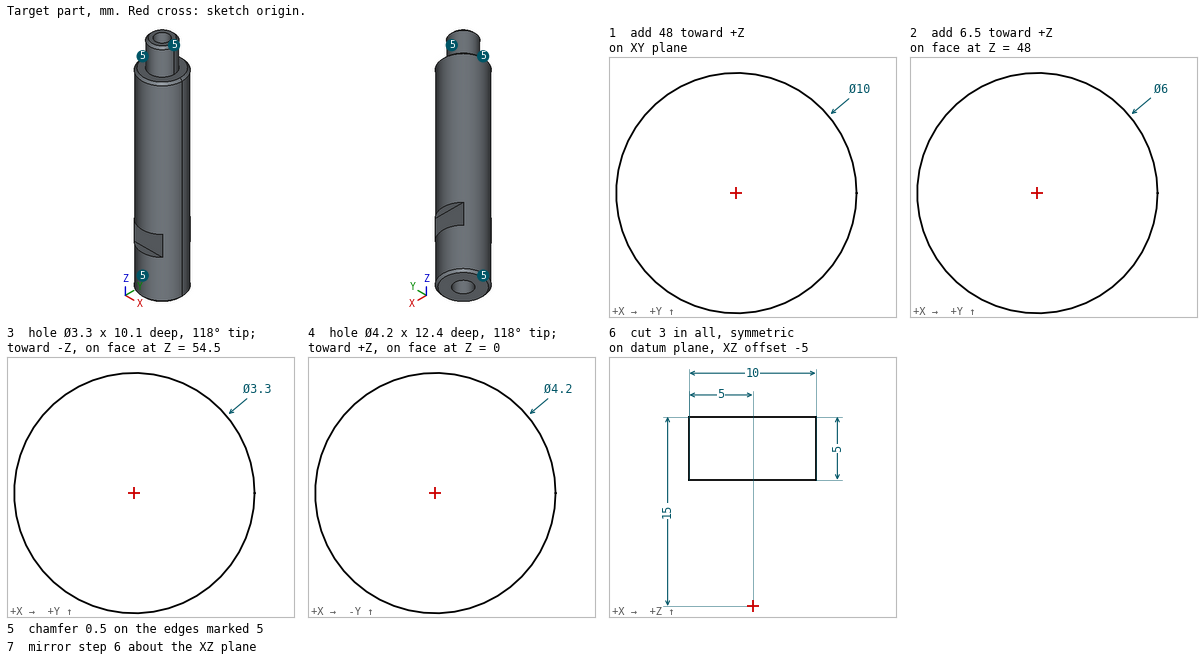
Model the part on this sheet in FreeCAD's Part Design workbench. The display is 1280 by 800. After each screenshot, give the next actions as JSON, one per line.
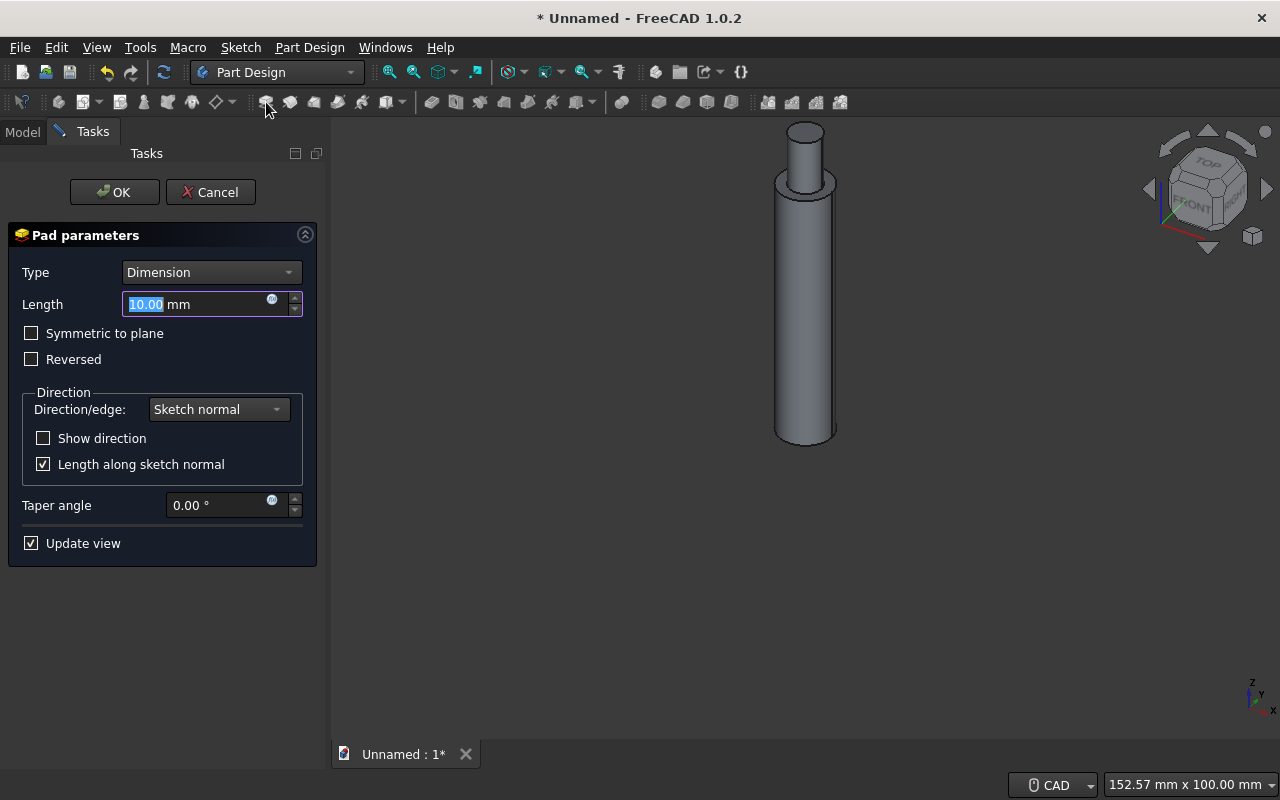
{"action": "type", "text": "6.5"}
{"action": "key", "text": "Tab"}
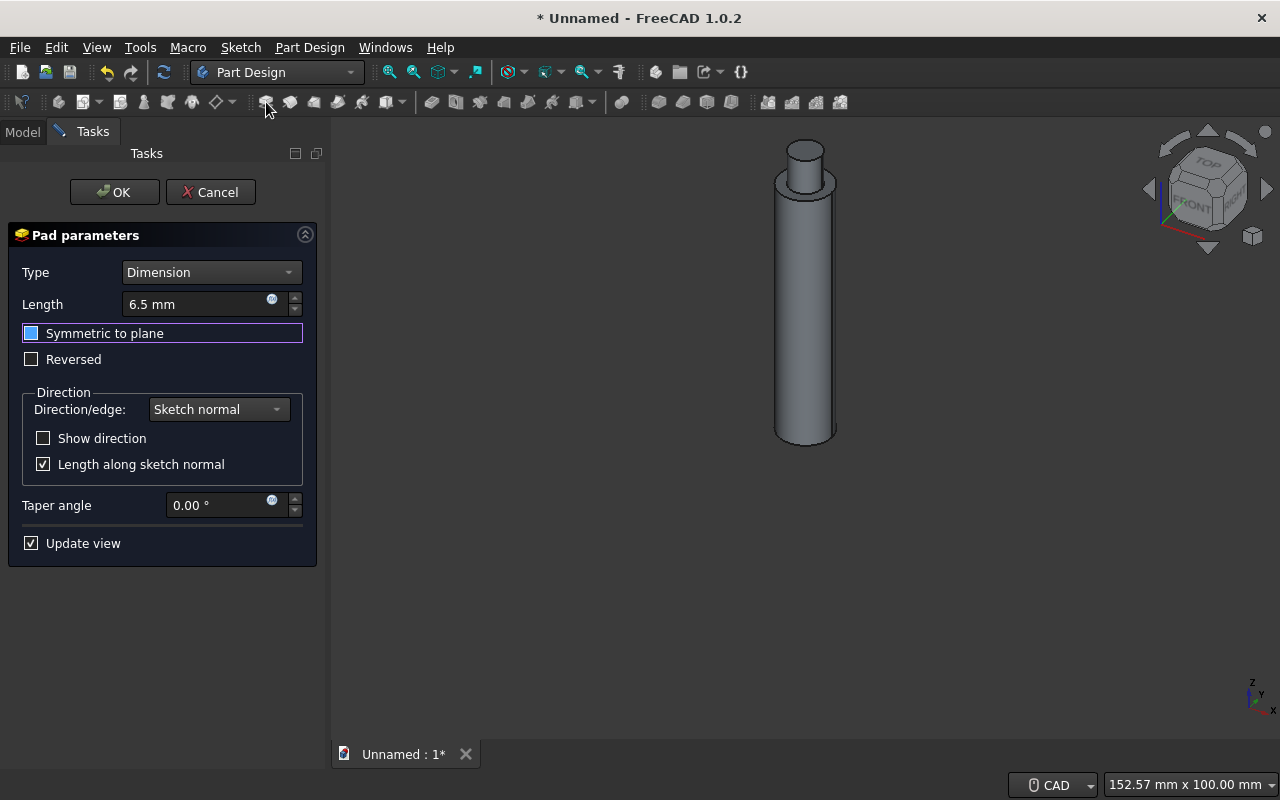
{"action": "left_click", "coordinate": [115, 192]}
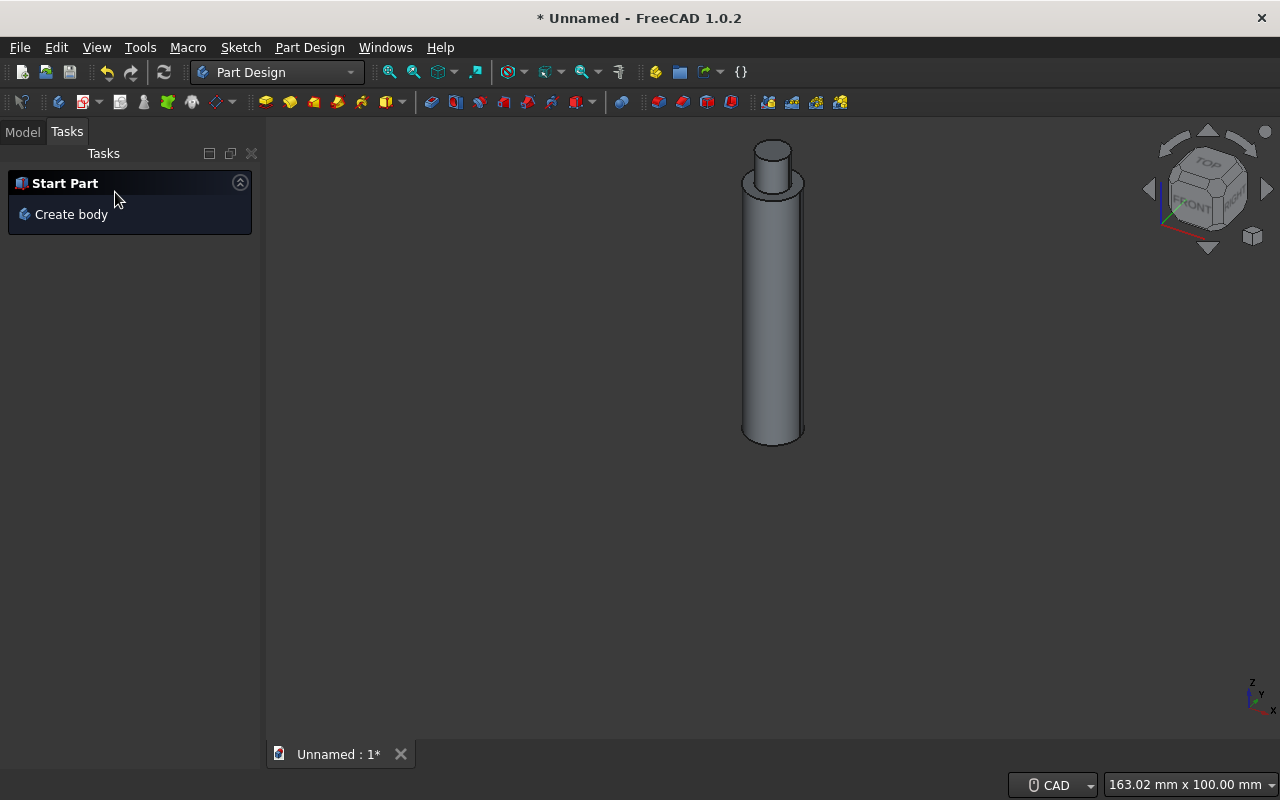
{"action": "left_click", "coordinate": [773, 149]}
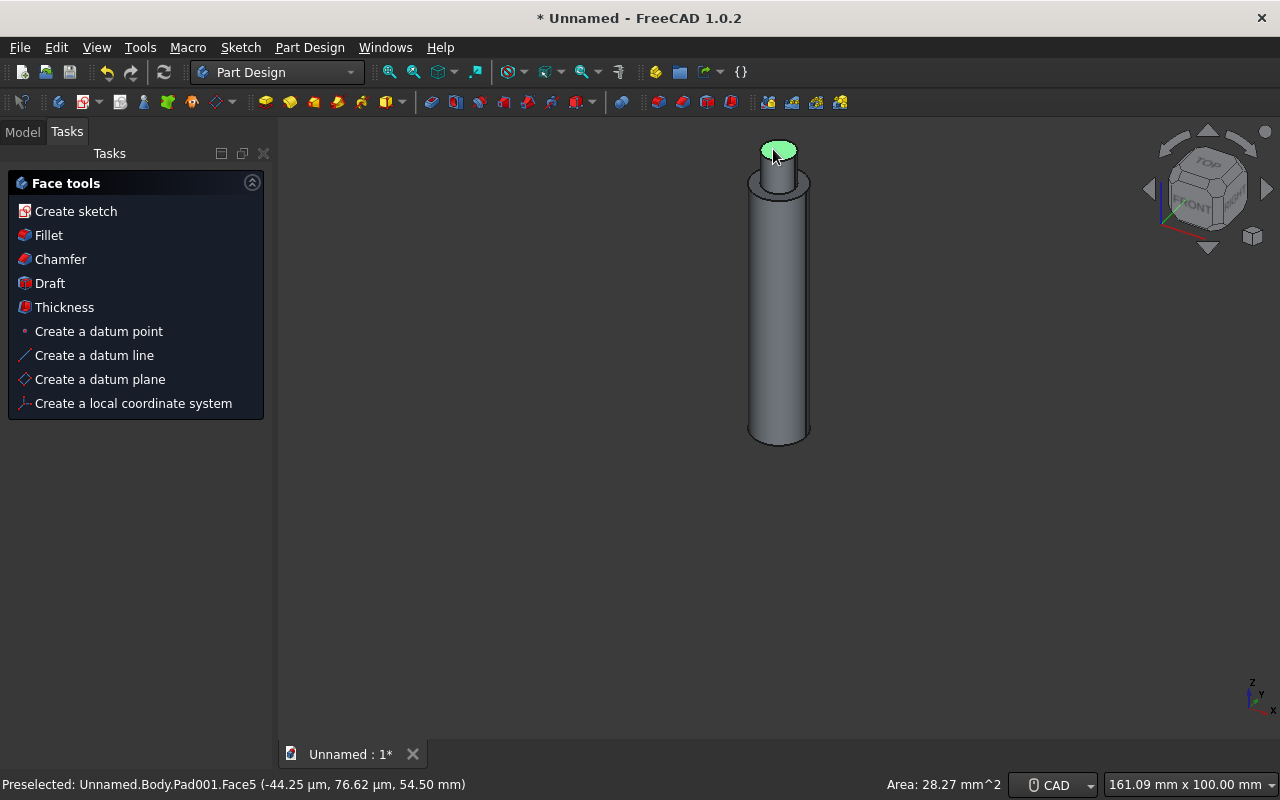
{"action": "left_click", "coordinate": [84, 102]}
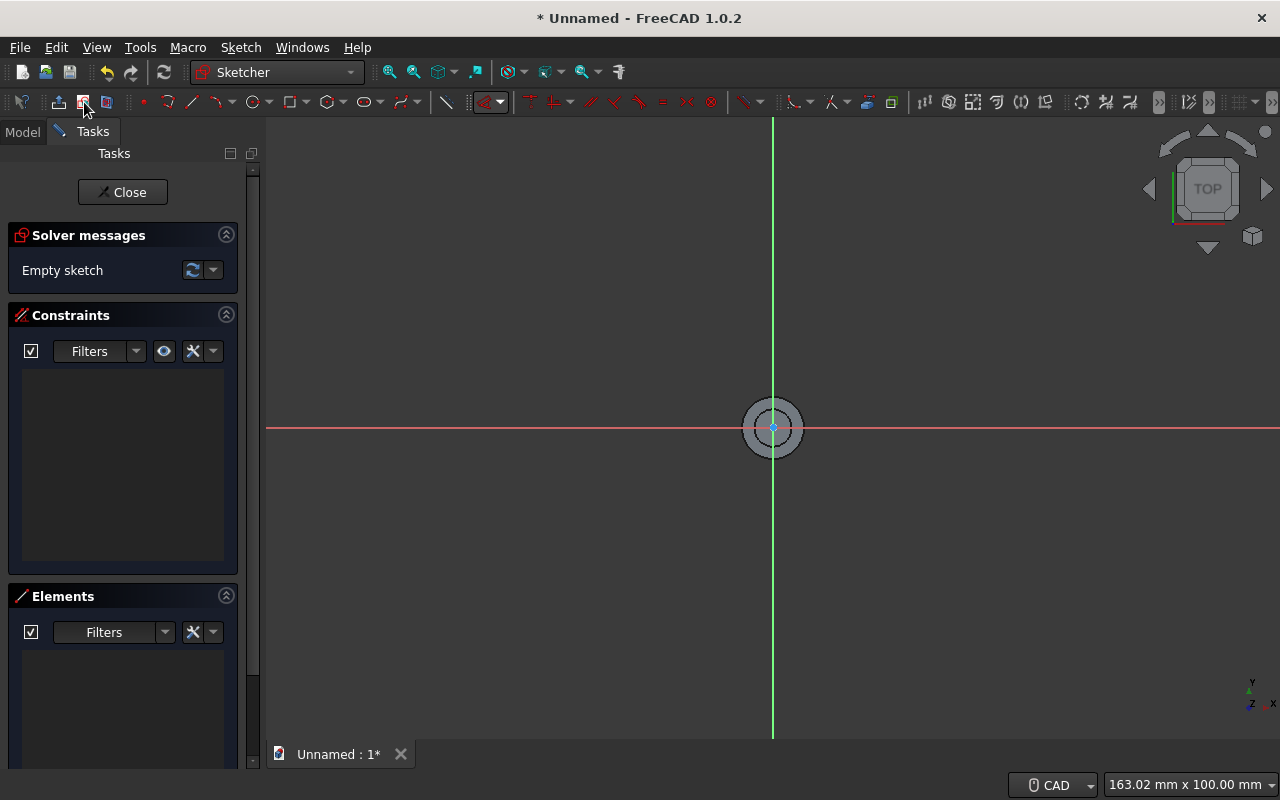
{"action": "scroll", "coordinate": [777, 428], "scroll_direction": "up", "scroll_amount": 15}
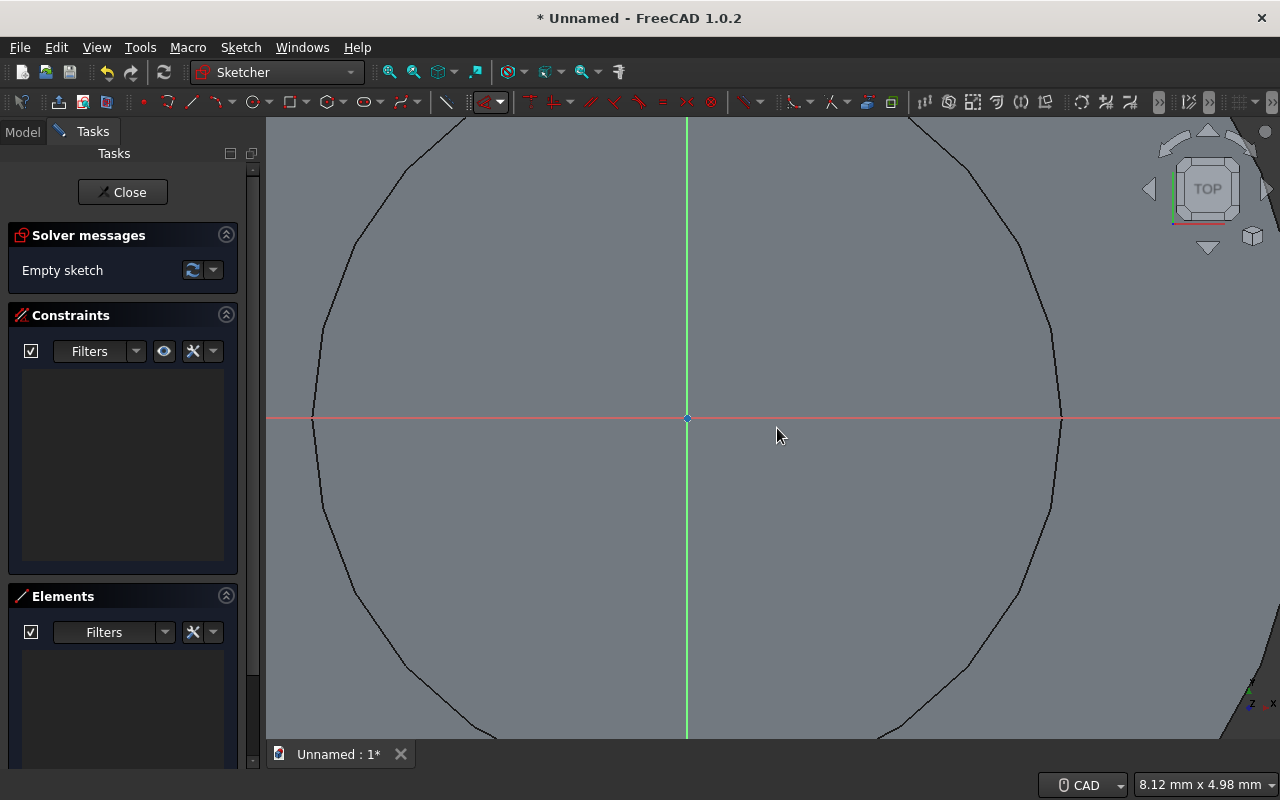
{"action": "left_click", "coordinate": [254, 102]}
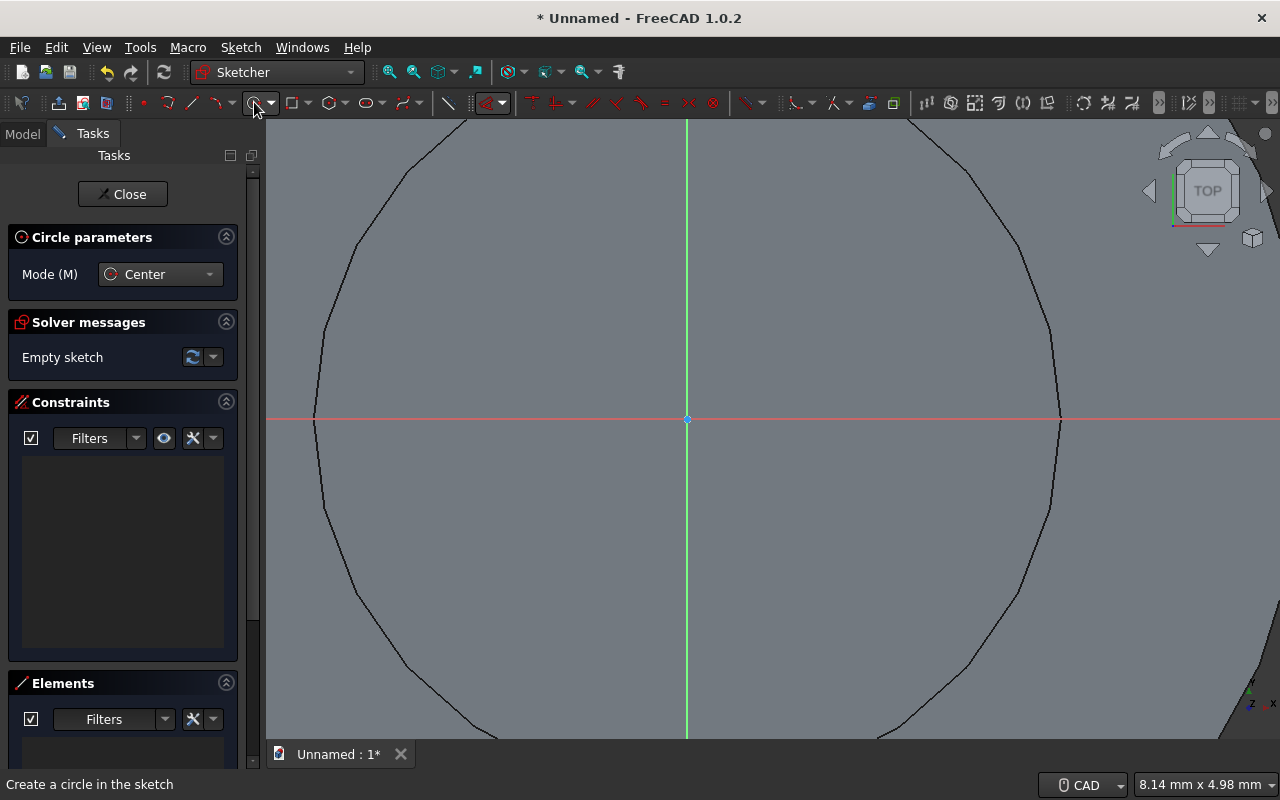
{"action": "left_click", "coordinate": [687, 419]}
{"action": "mouse_move", "coordinate": [833, 274]}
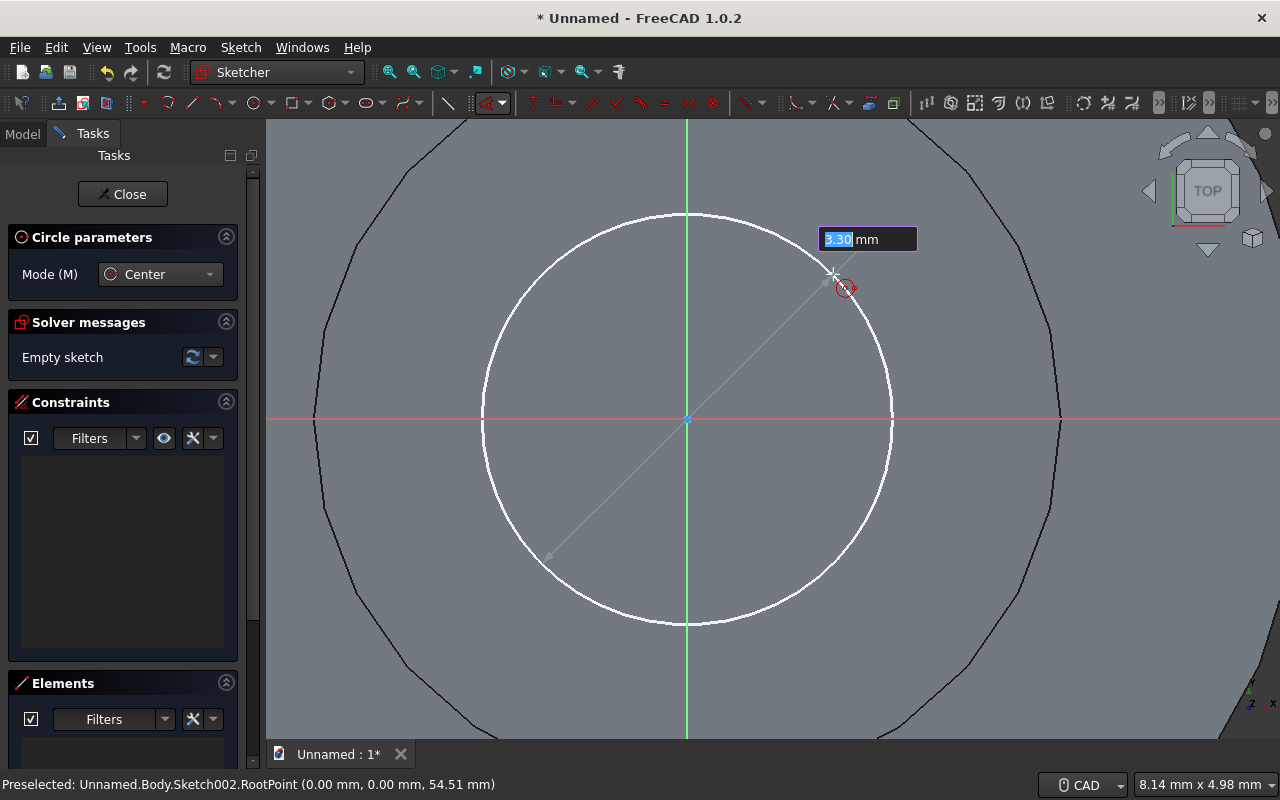
{"action": "type", "text": "3.3"}
{"action": "key", "text": "Return"}
{"action": "key", "text": "Escape"}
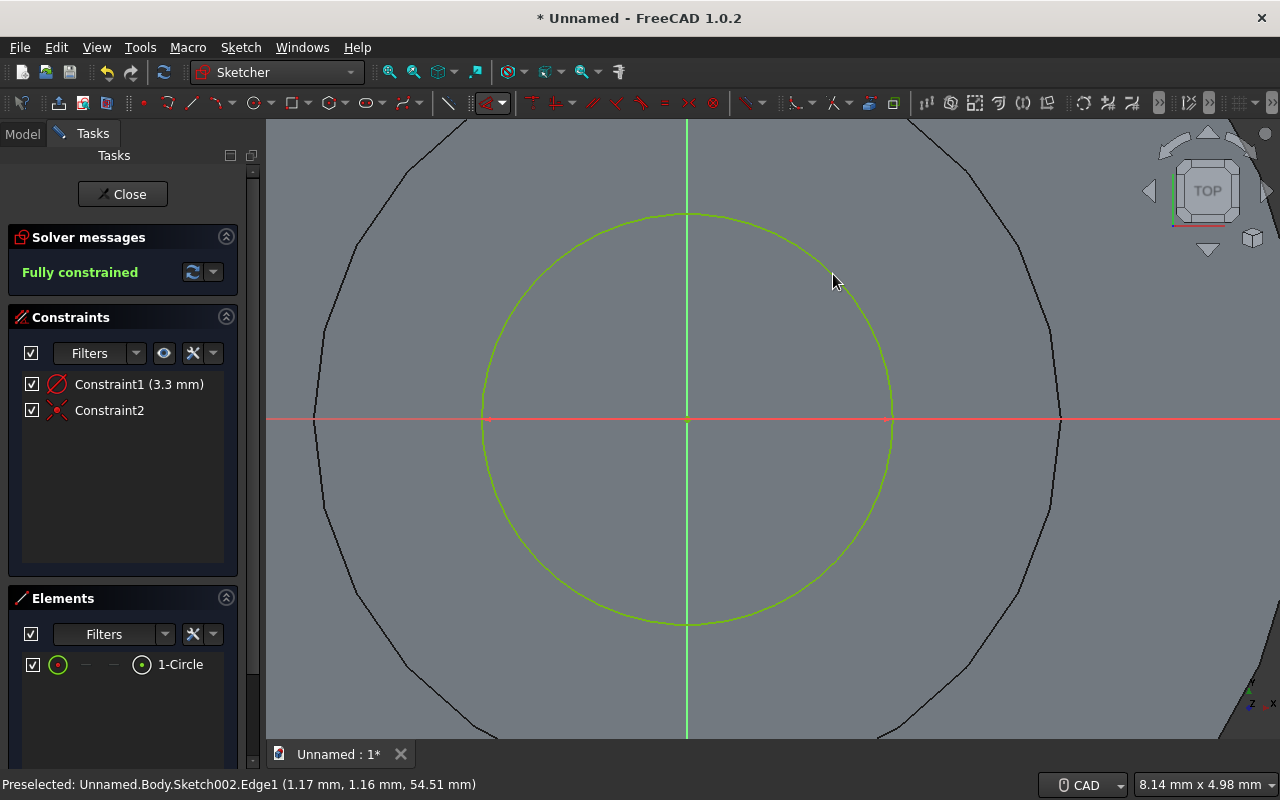
{"action": "left_click", "coordinate": [123, 194]}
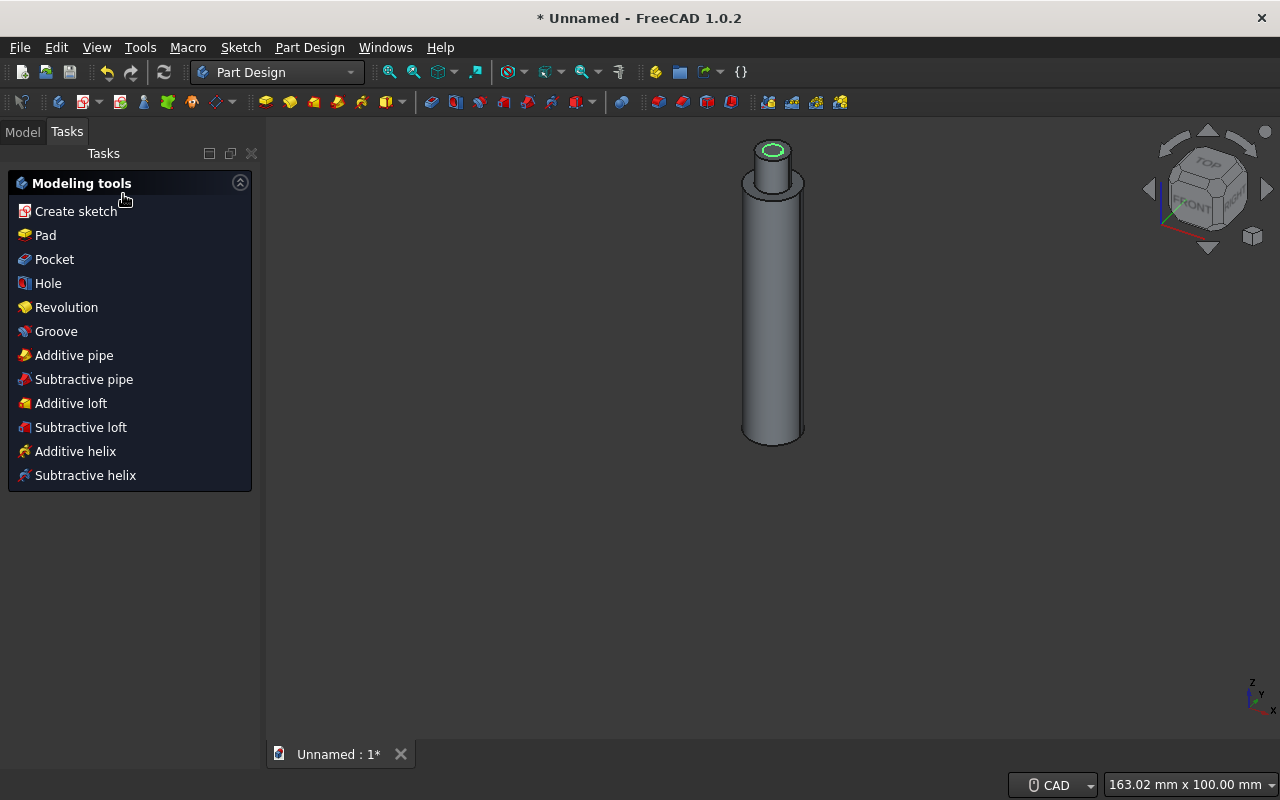
{"action": "left_click", "coordinate": [456, 102]}